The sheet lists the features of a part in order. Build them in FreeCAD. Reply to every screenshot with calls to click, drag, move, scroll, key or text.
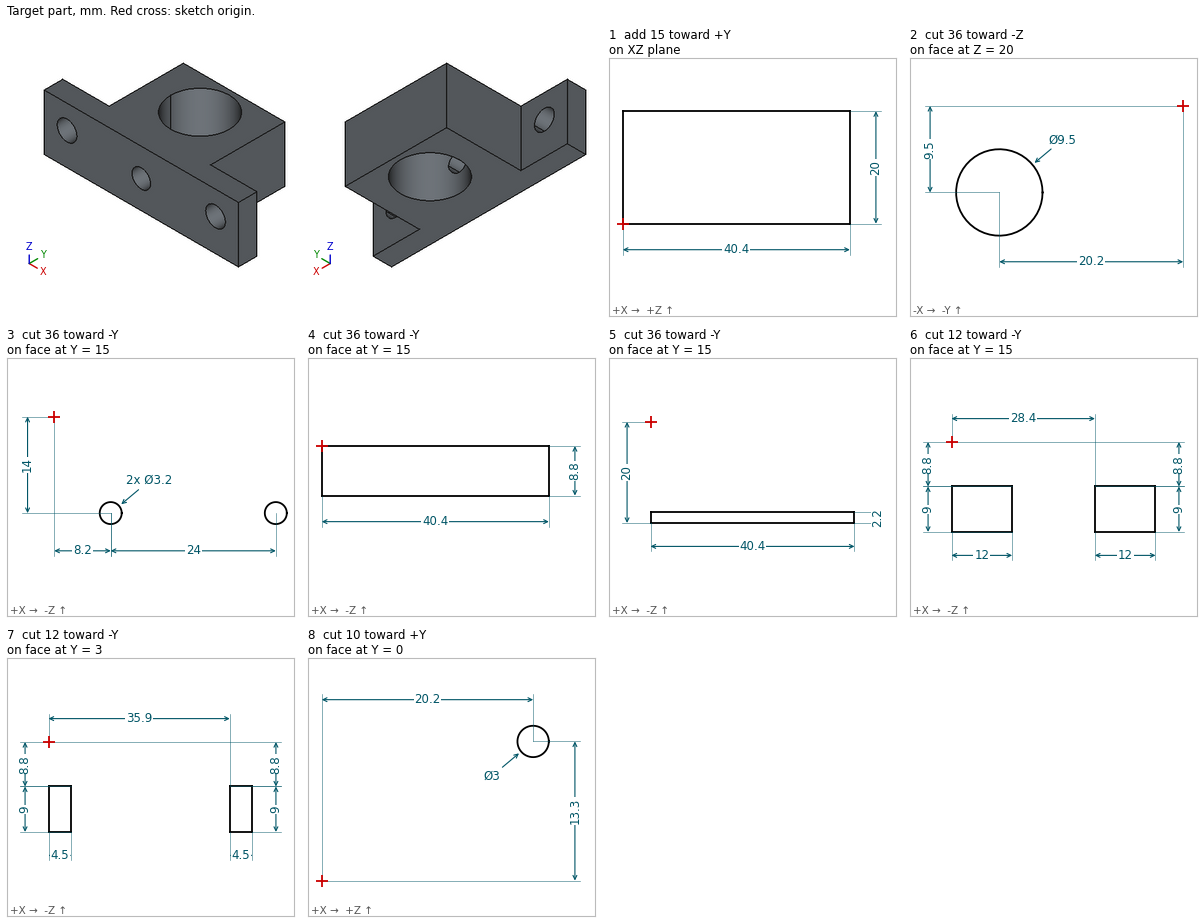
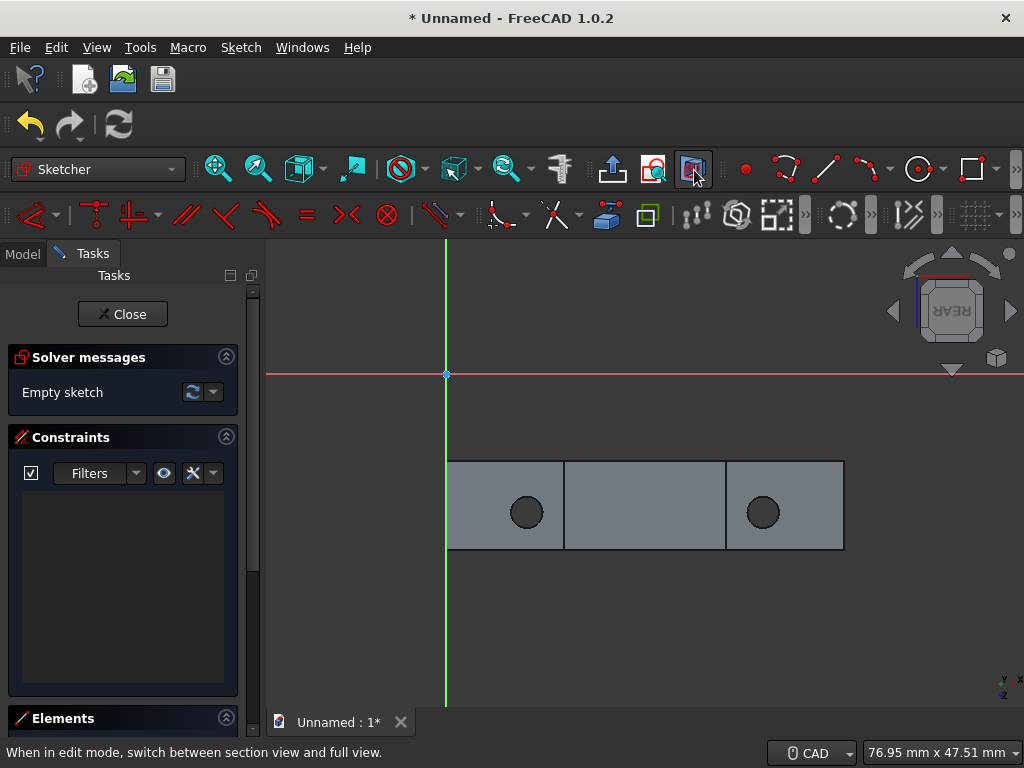
scroll(294, 522, down, 1)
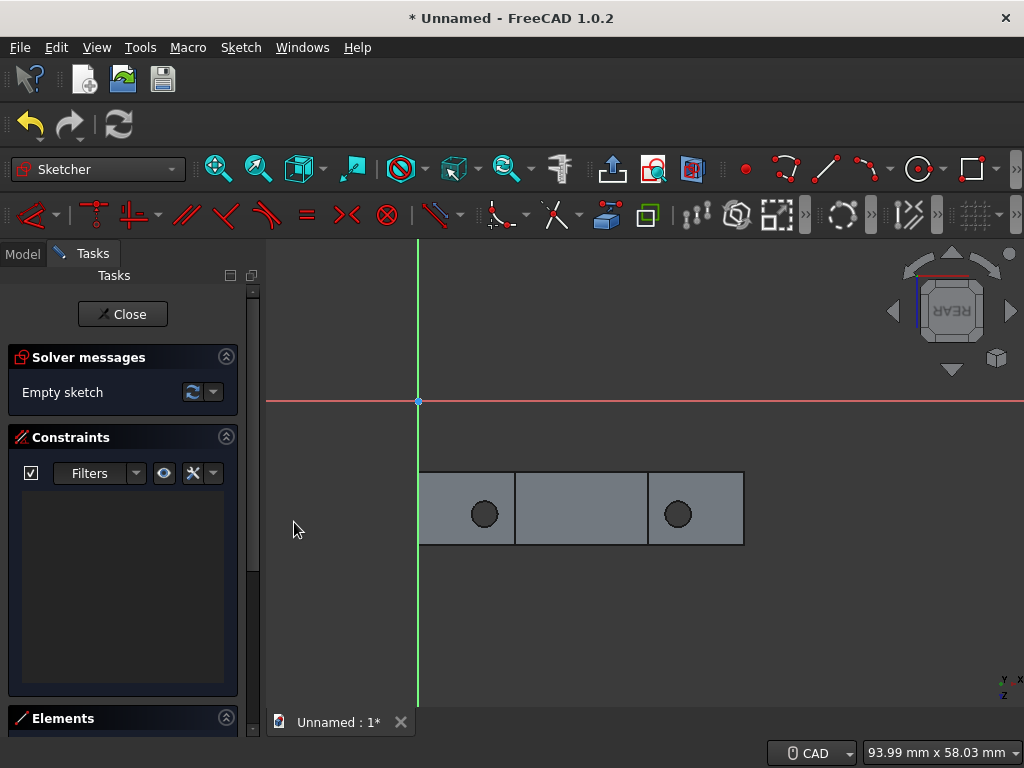
key(g)
key(r)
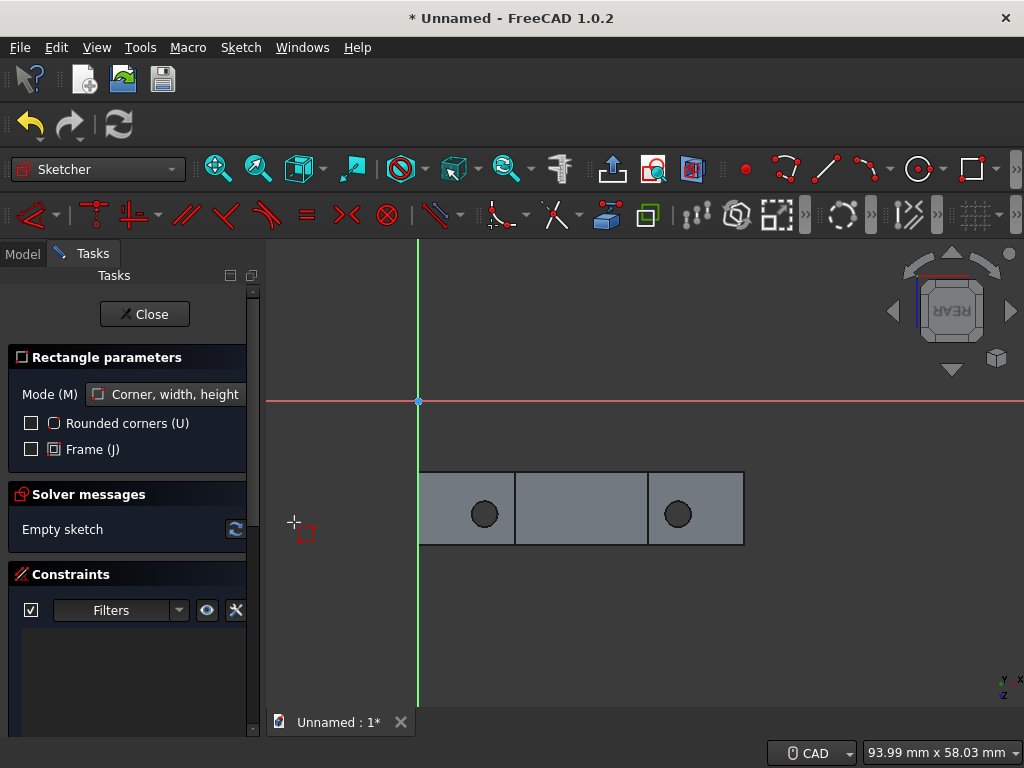
click(418, 472)
move(455, 545)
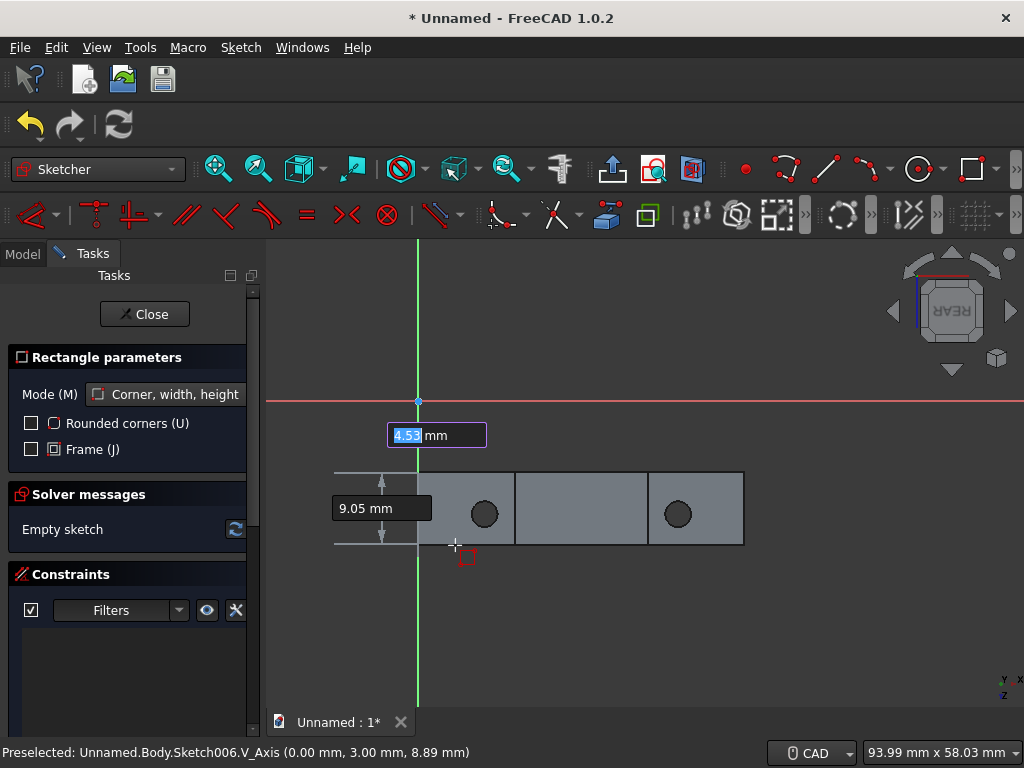
text(4.5)
key(Tab)
text(9)
key(Return)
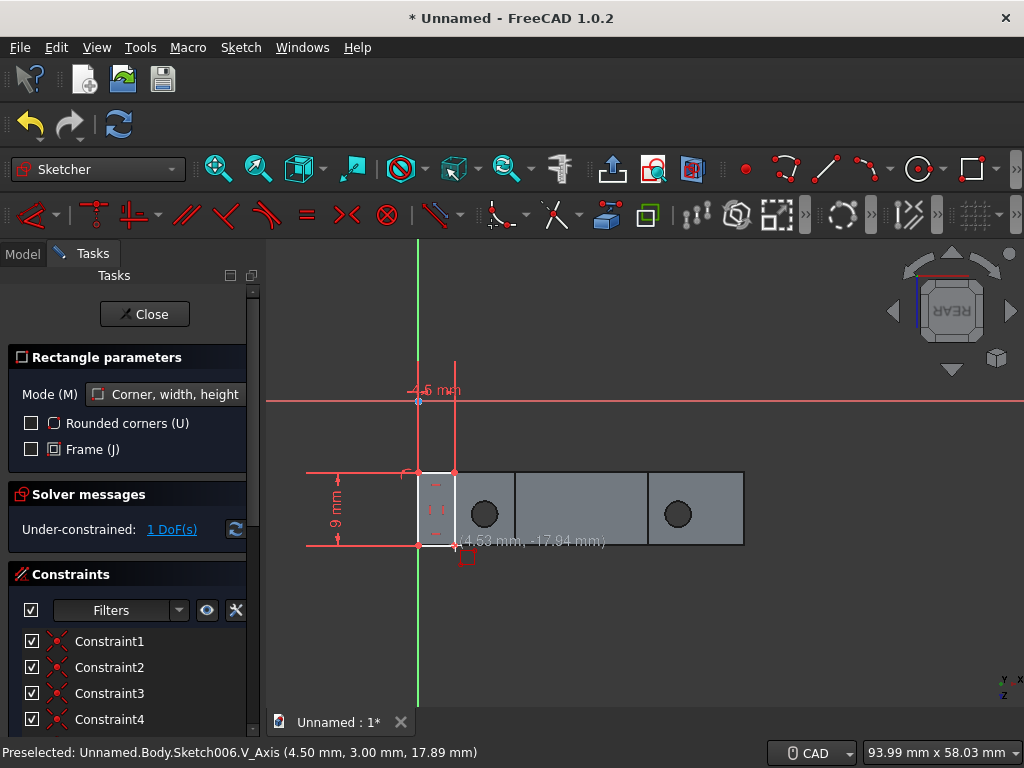
click(708, 472)
move(744, 545)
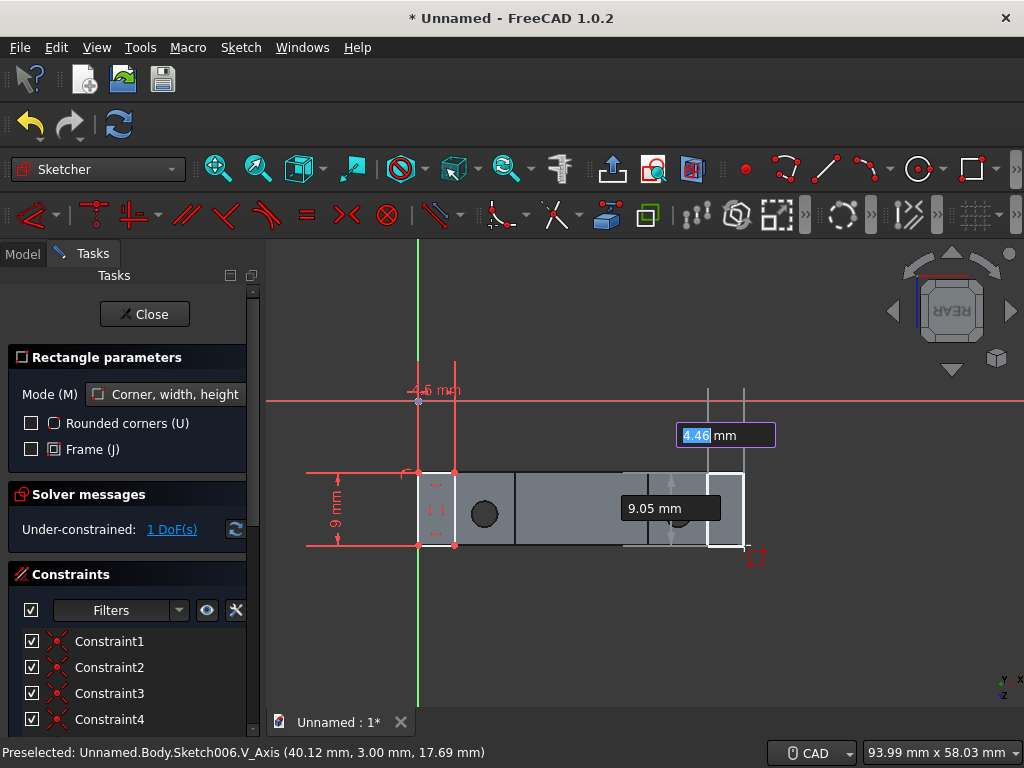
text(4.5)
key(Tab)
text(9)
key(Return)
key(Escape)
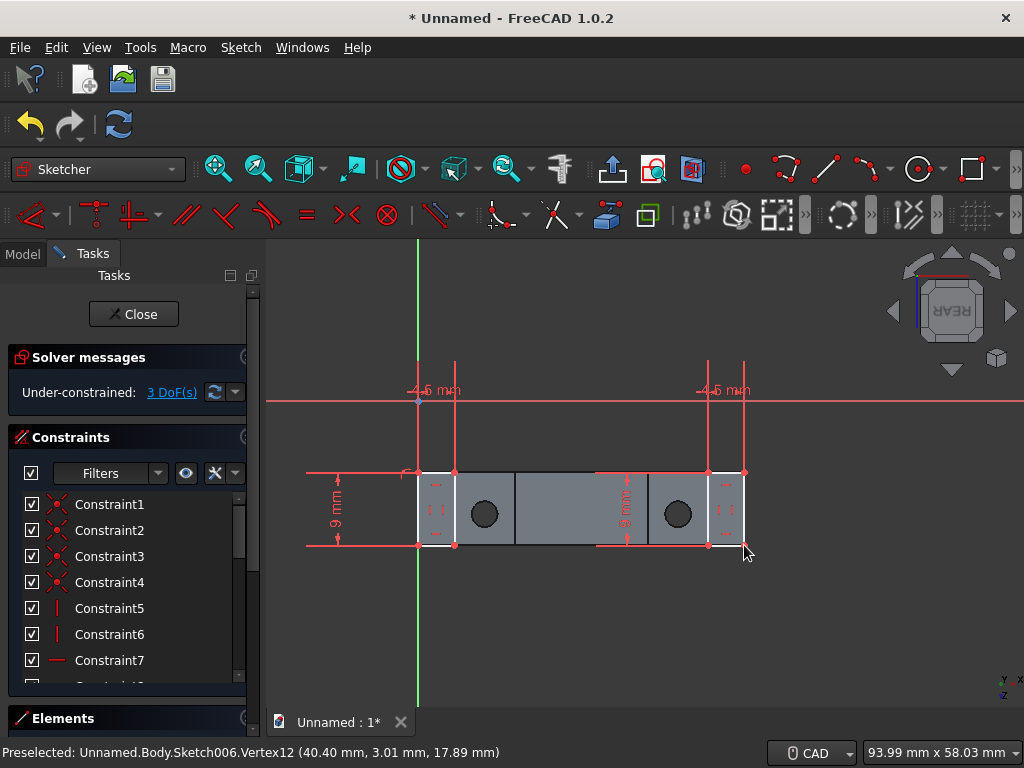
click(418, 473)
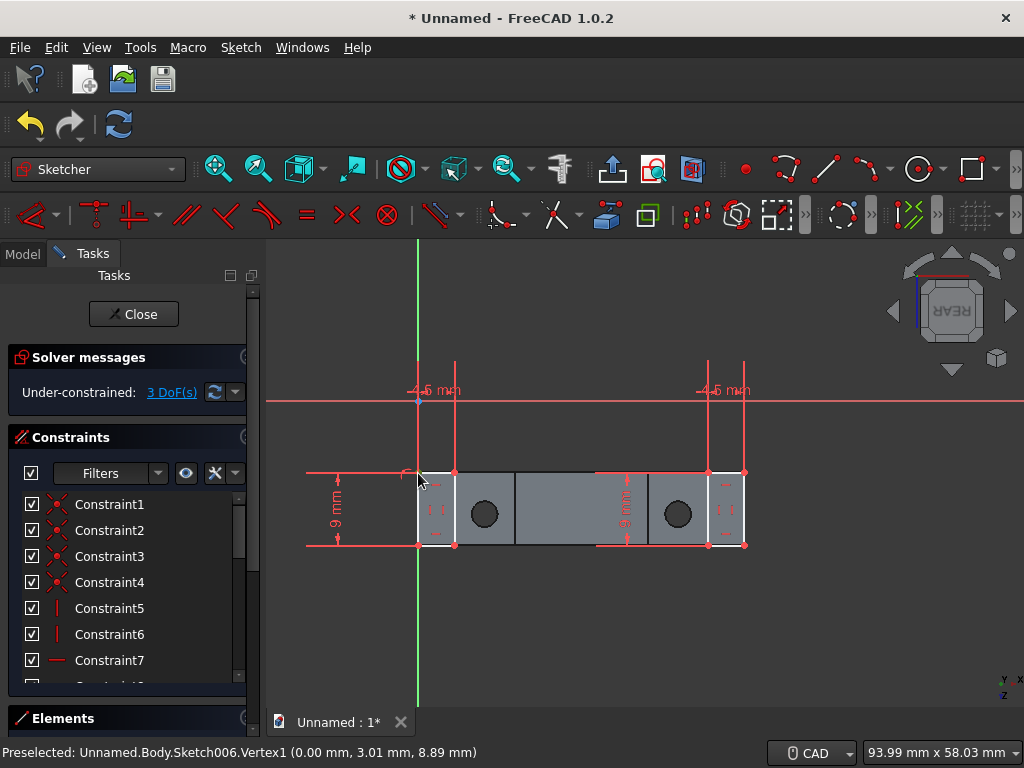
key(i)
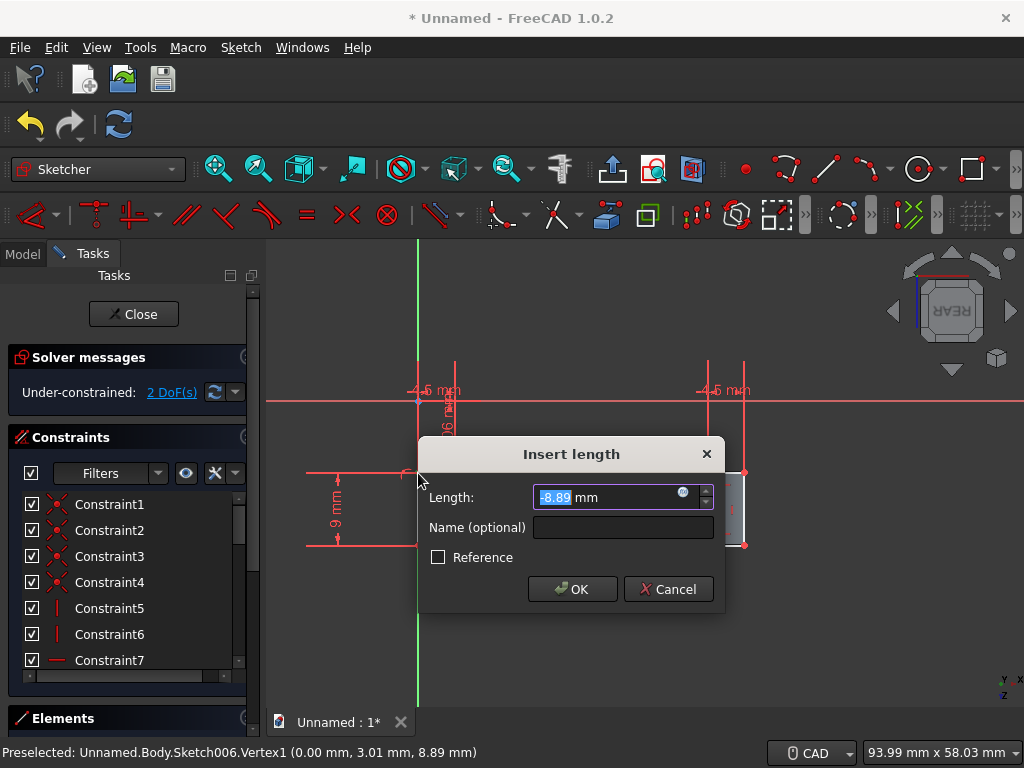
text(-8.8)
key(Return)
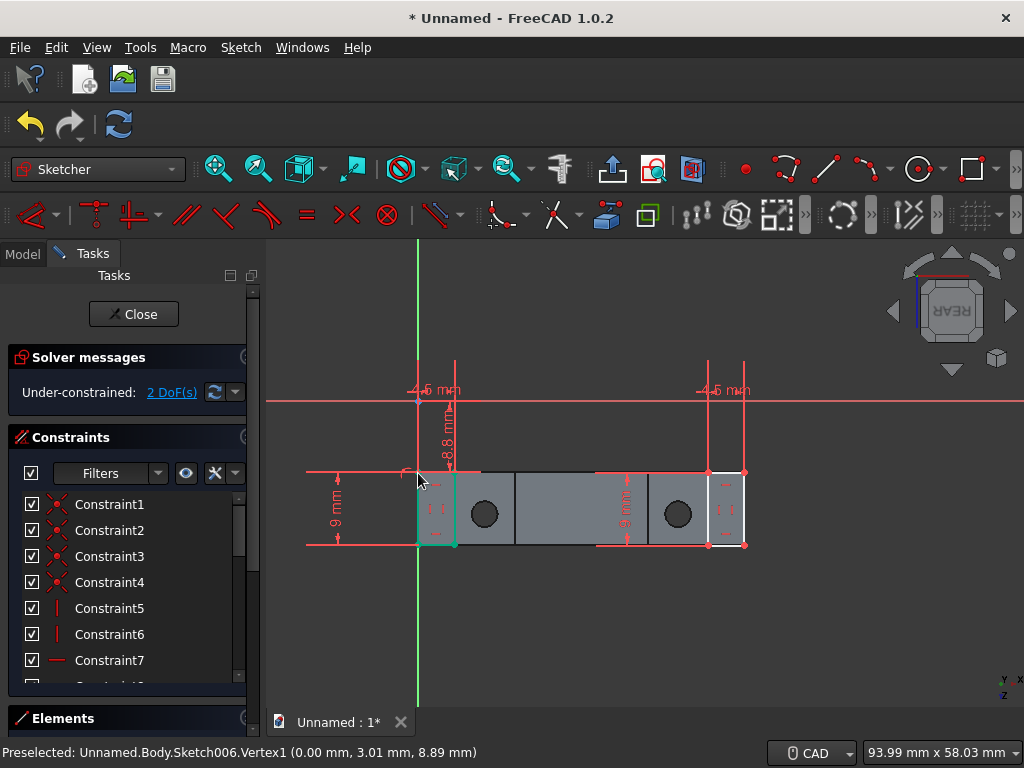
click(708, 473)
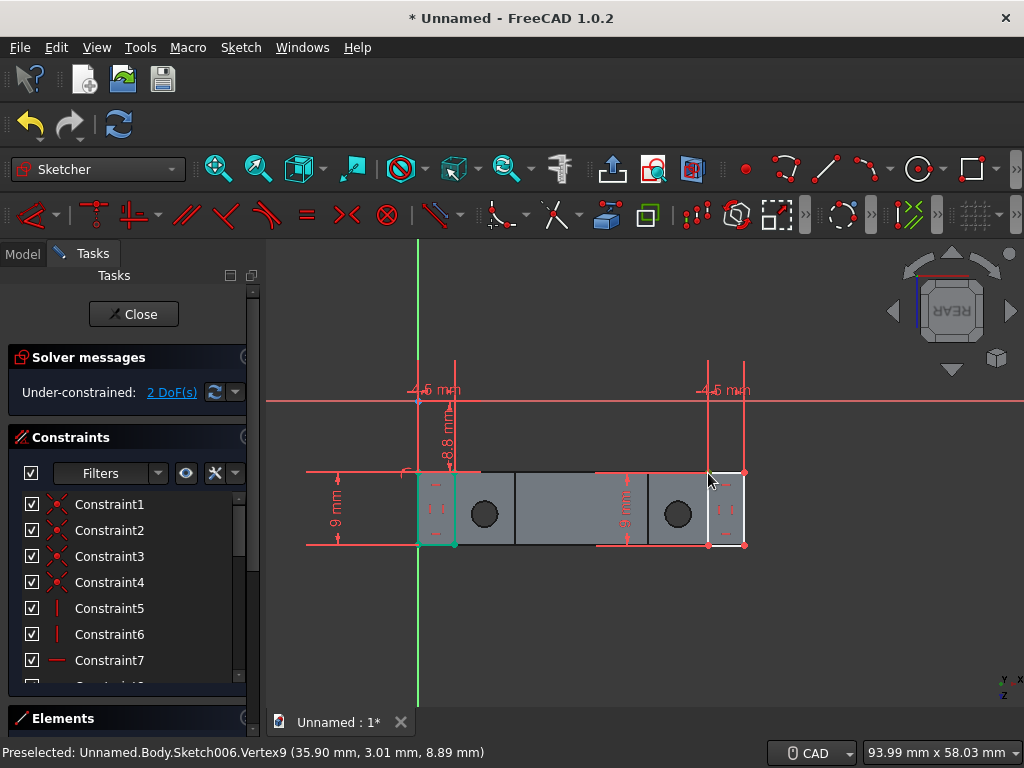
key(i)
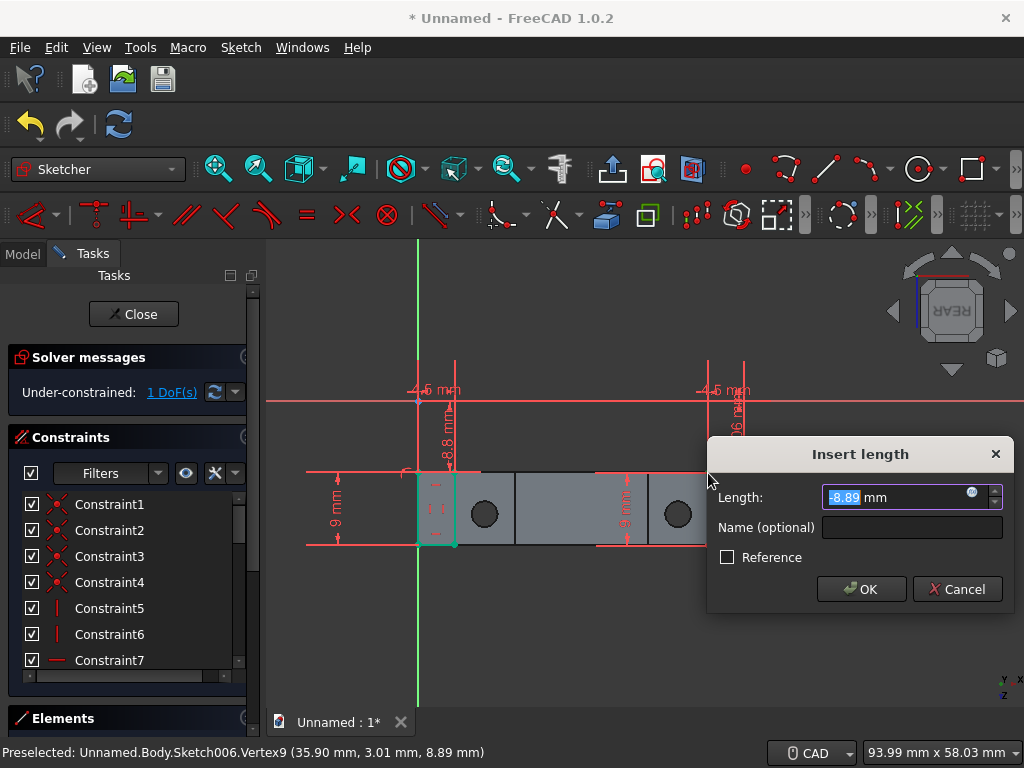
text(-8.8)
key(Return)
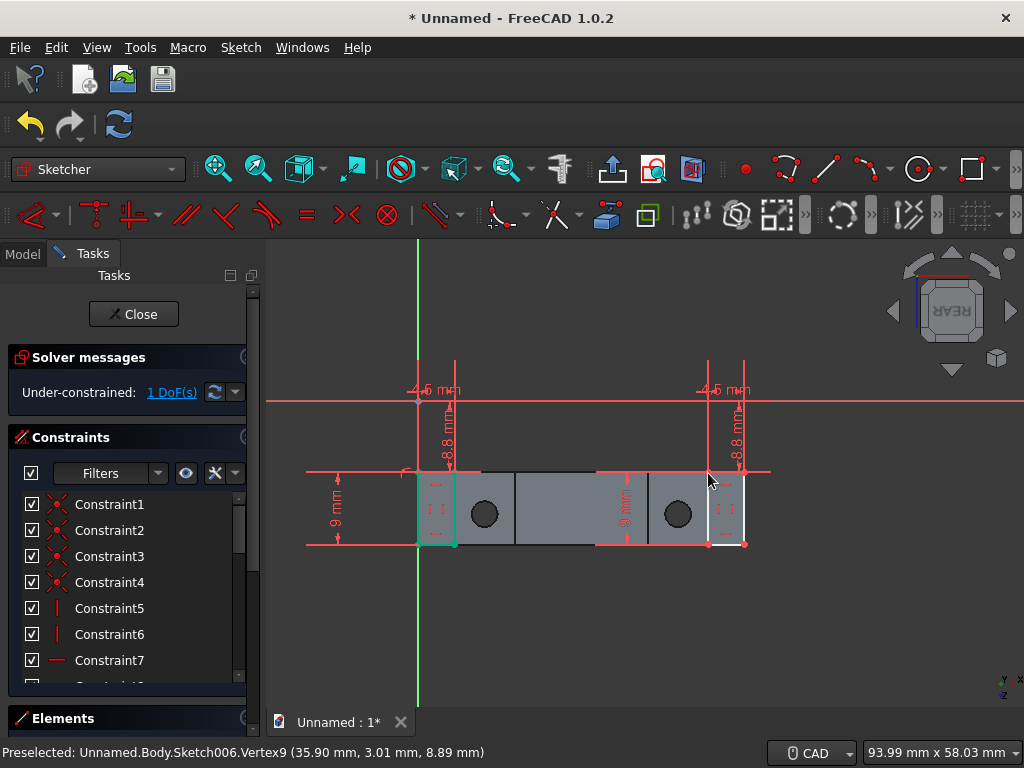
click(708, 472)